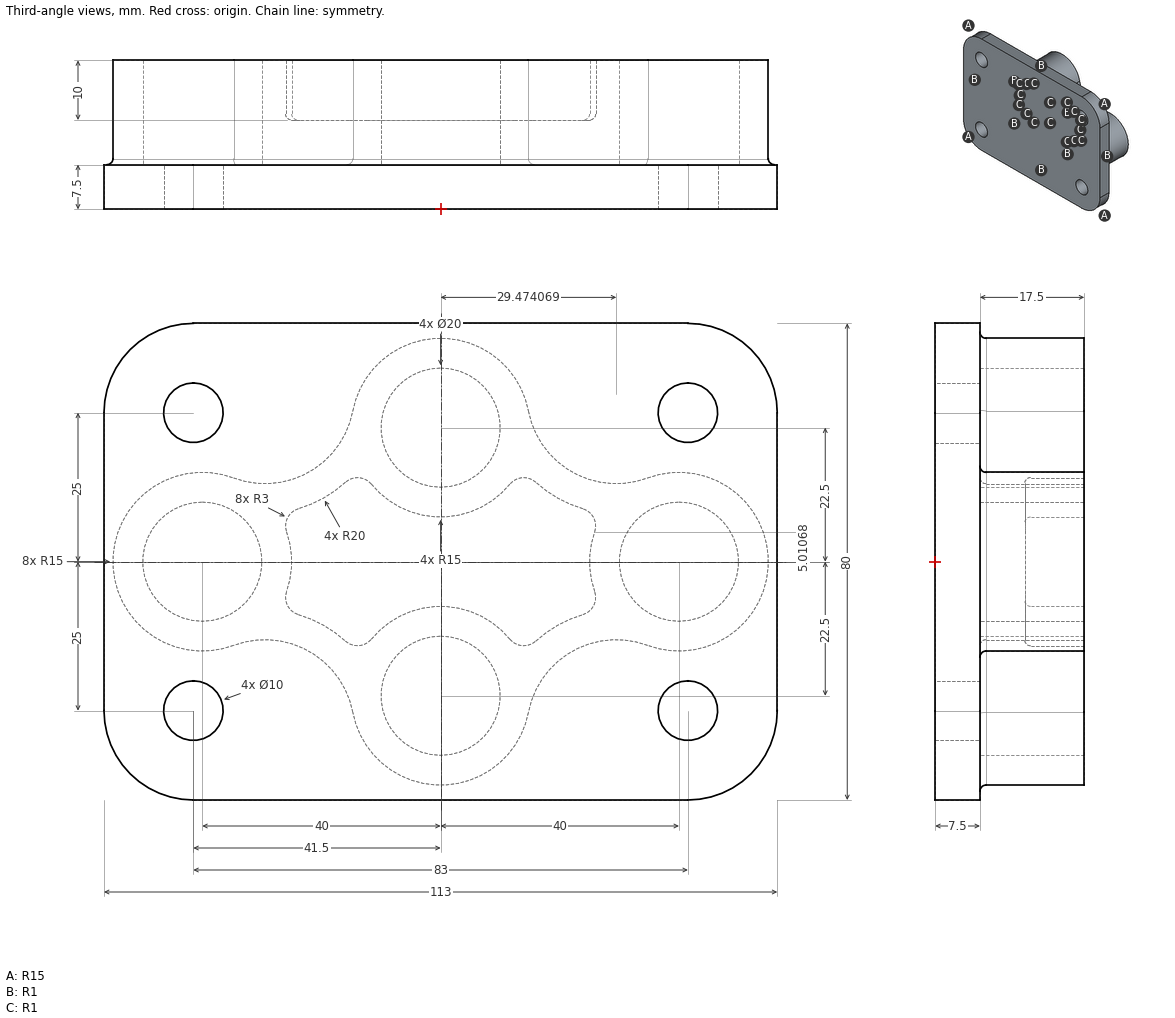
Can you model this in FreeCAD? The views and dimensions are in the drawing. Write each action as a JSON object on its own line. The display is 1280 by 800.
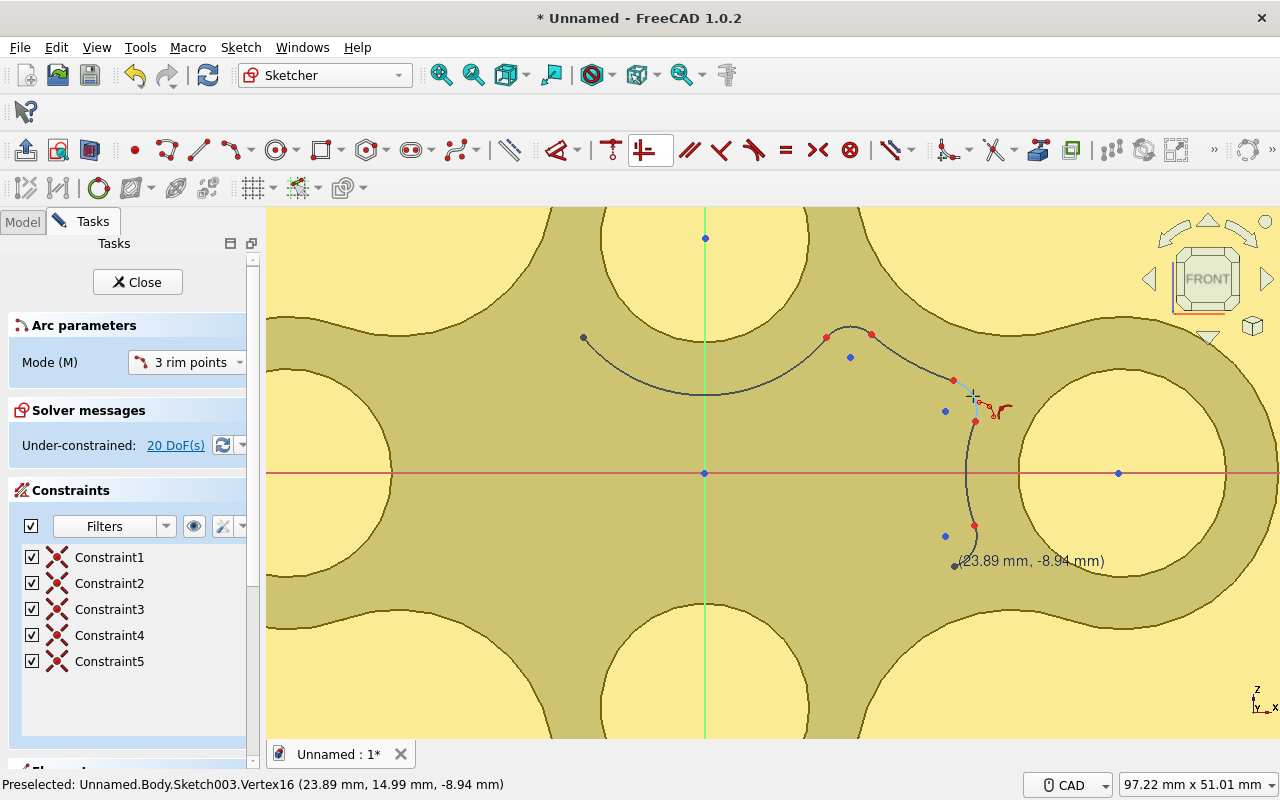
{"action": "left_click", "coordinate": [872, 612]}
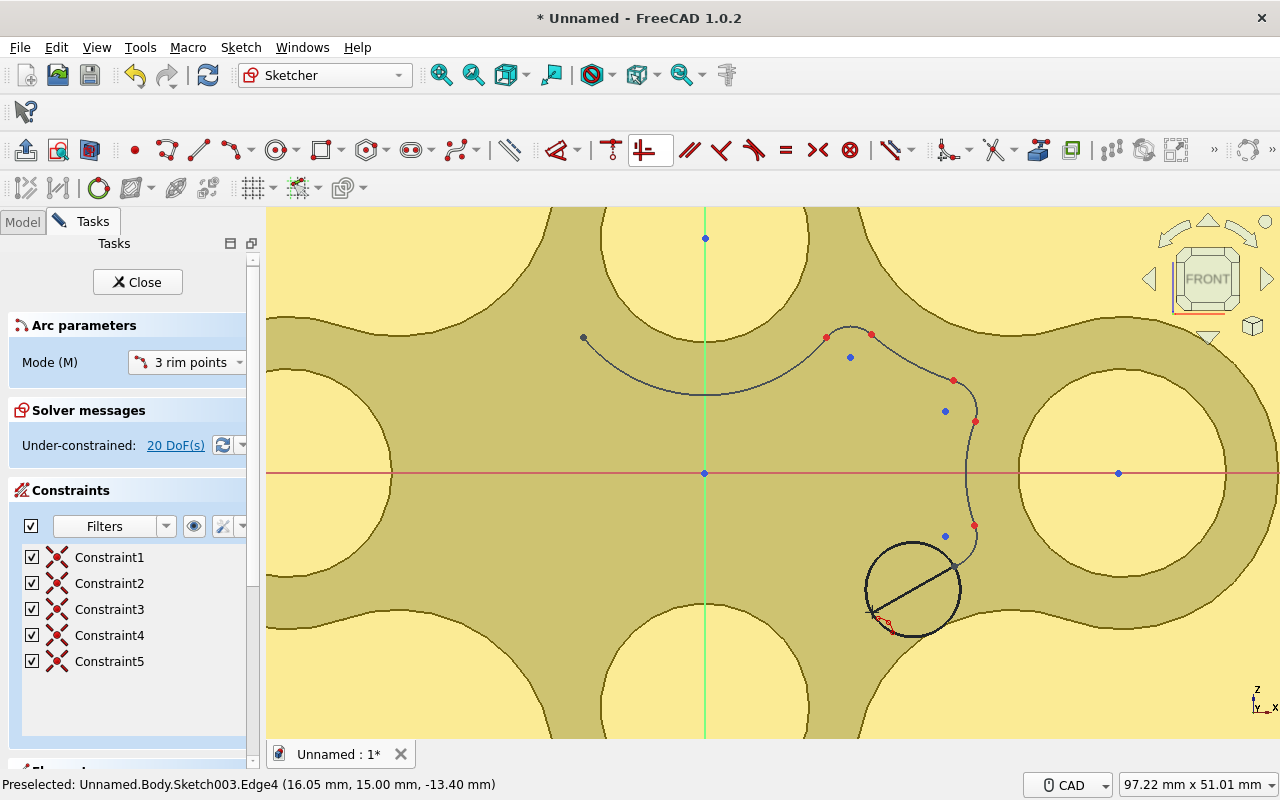
{"action": "scroll", "coordinate": [910, 584], "scroll_direction": "up", "scroll_amount": 6}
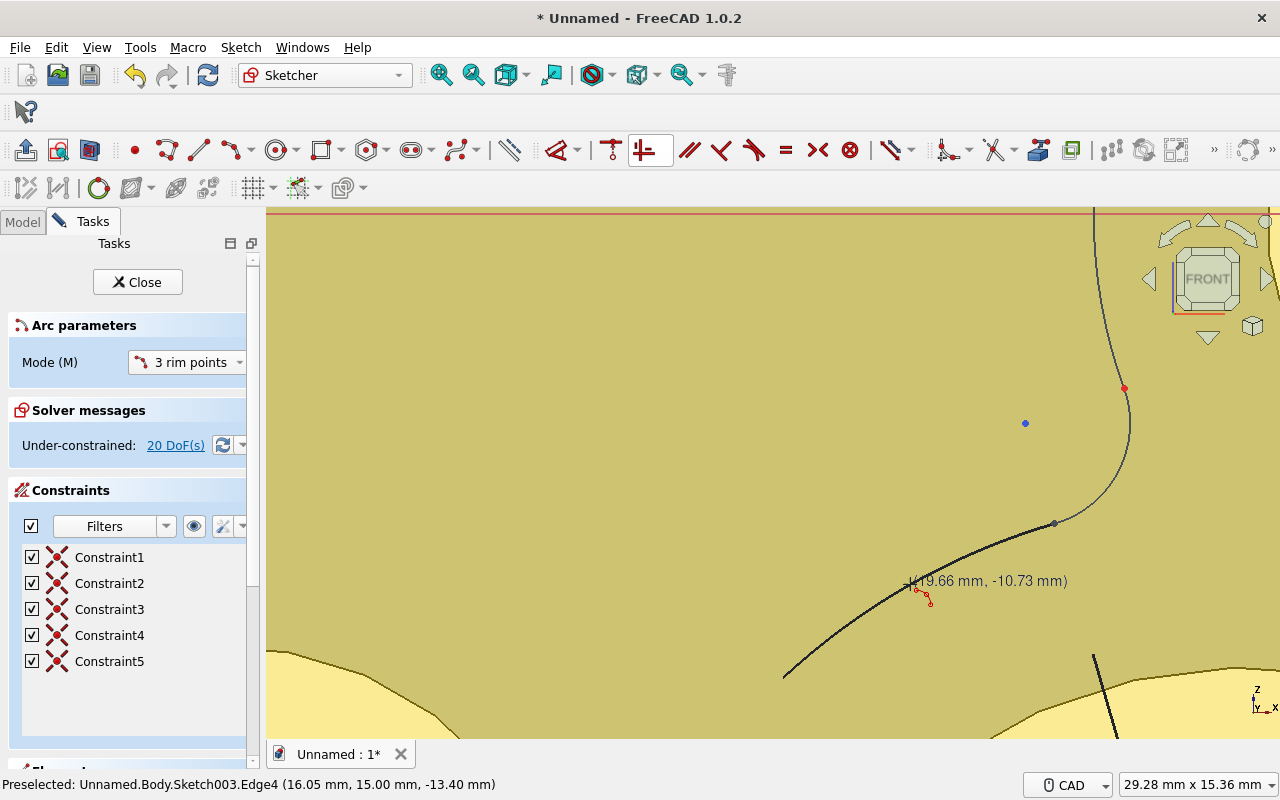
{"action": "left_click", "coordinate": [909, 583]}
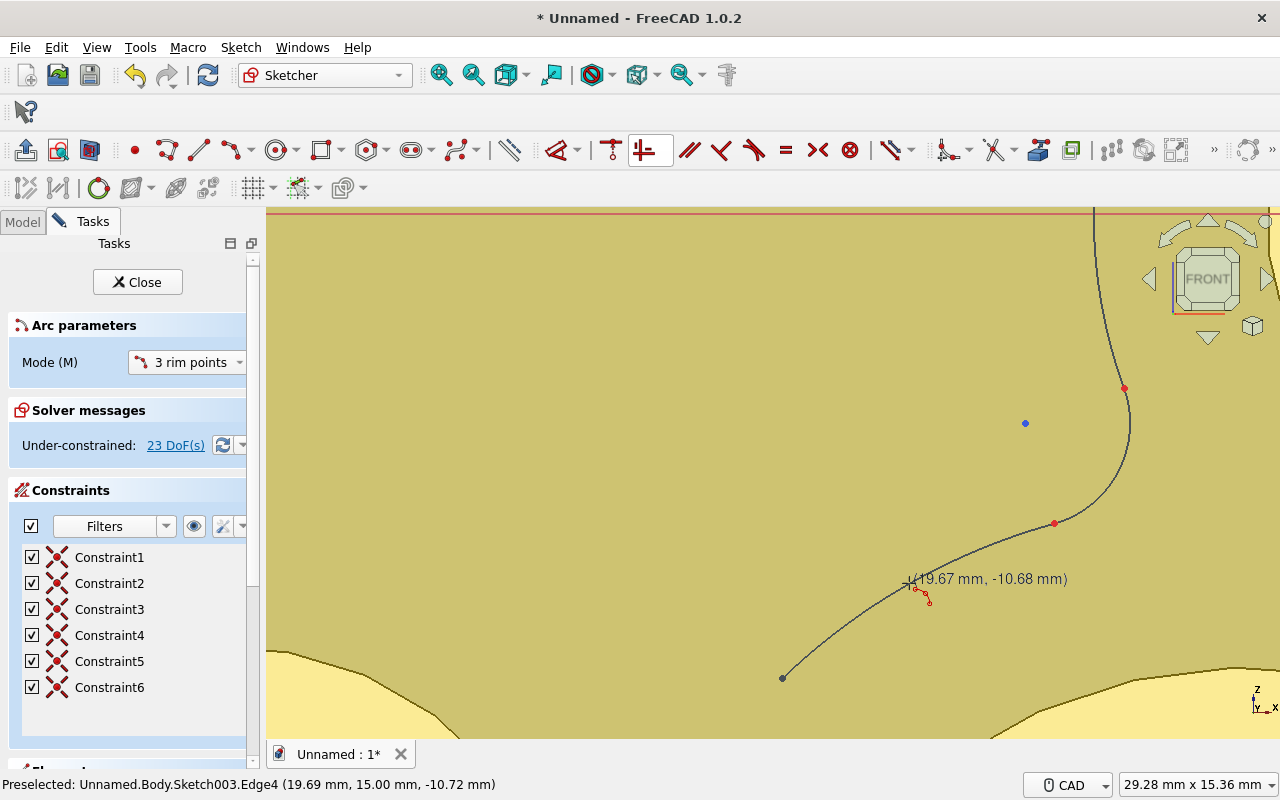
{"action": "left_click", "coordinate": [782, 679]}
{"action": "left_click", "coordinate": [630, 665]}
{"action": "left_click", "coordinate": [703, 703]}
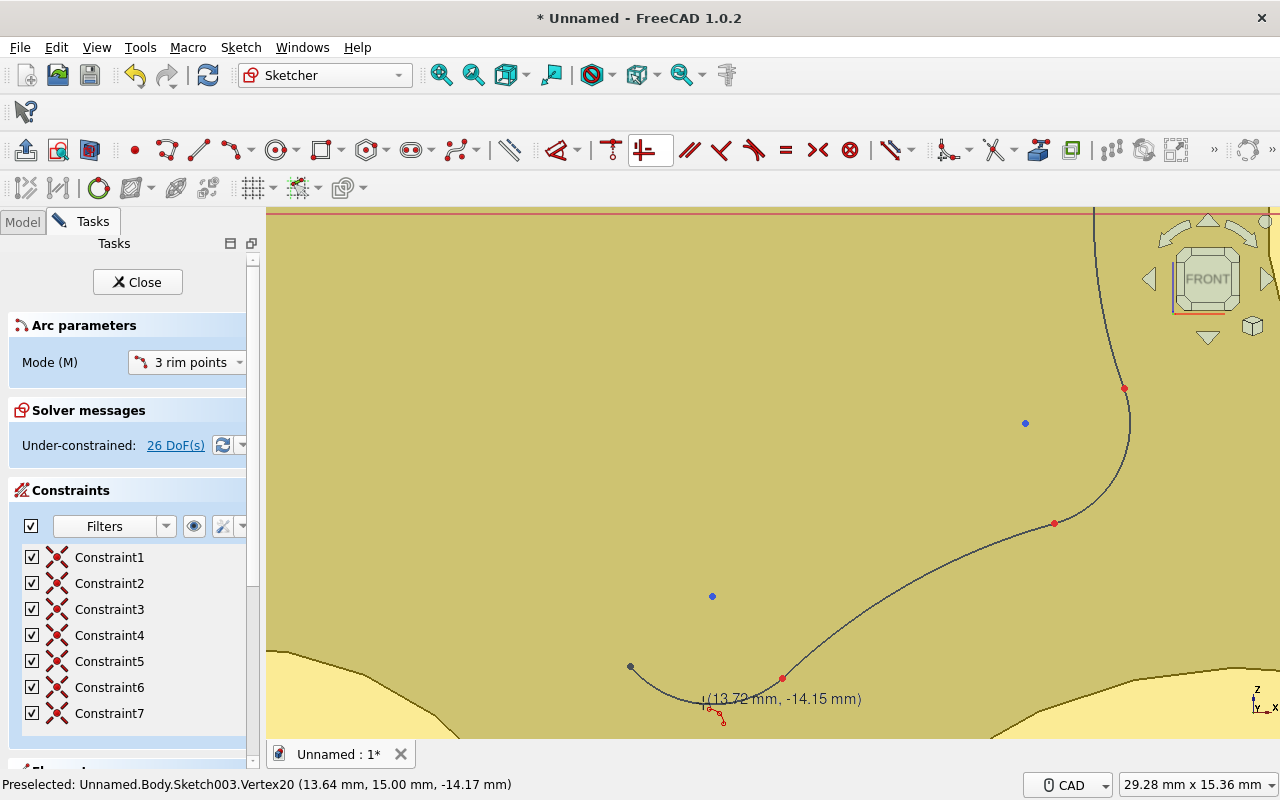
{"action": "left_click", "coordinate": [630, 666]}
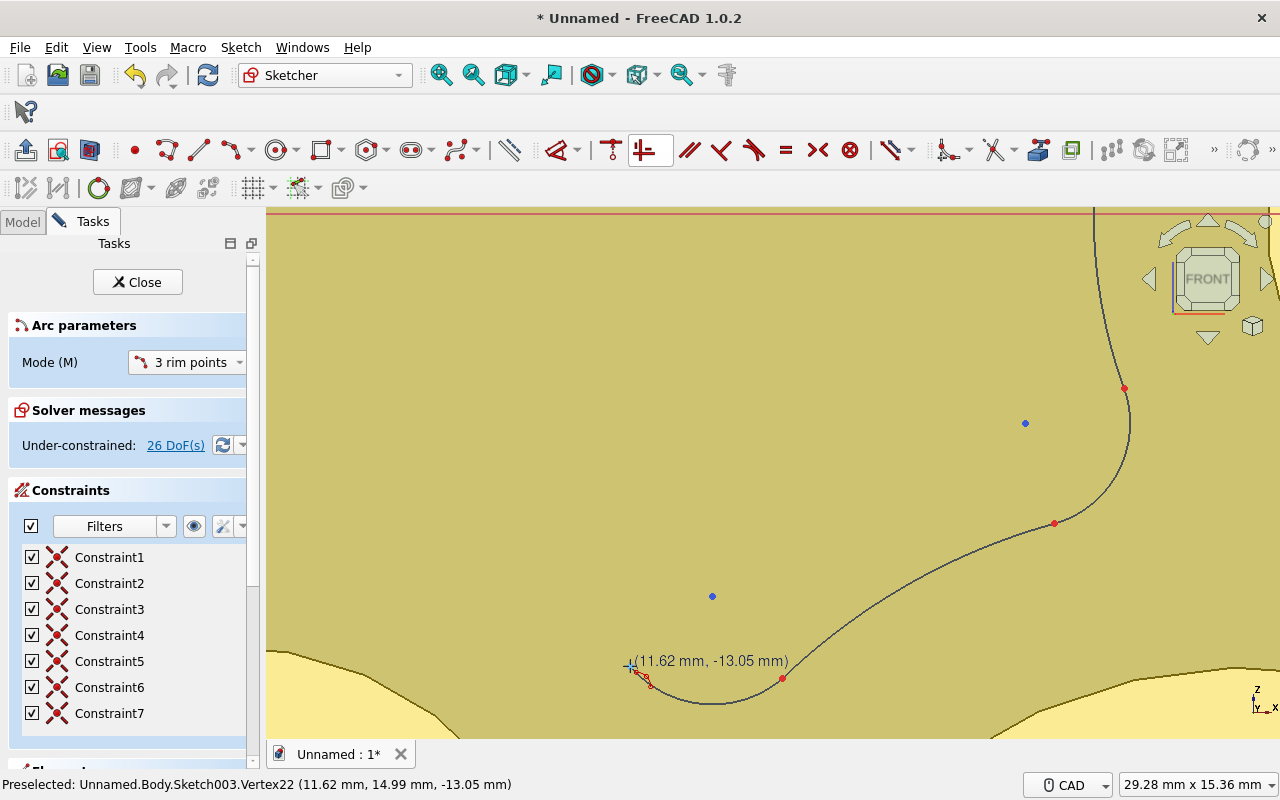
{"action": "scroll", "coordinate": [910, 585], "scroll_direction": "down", "scroll_amount": 6}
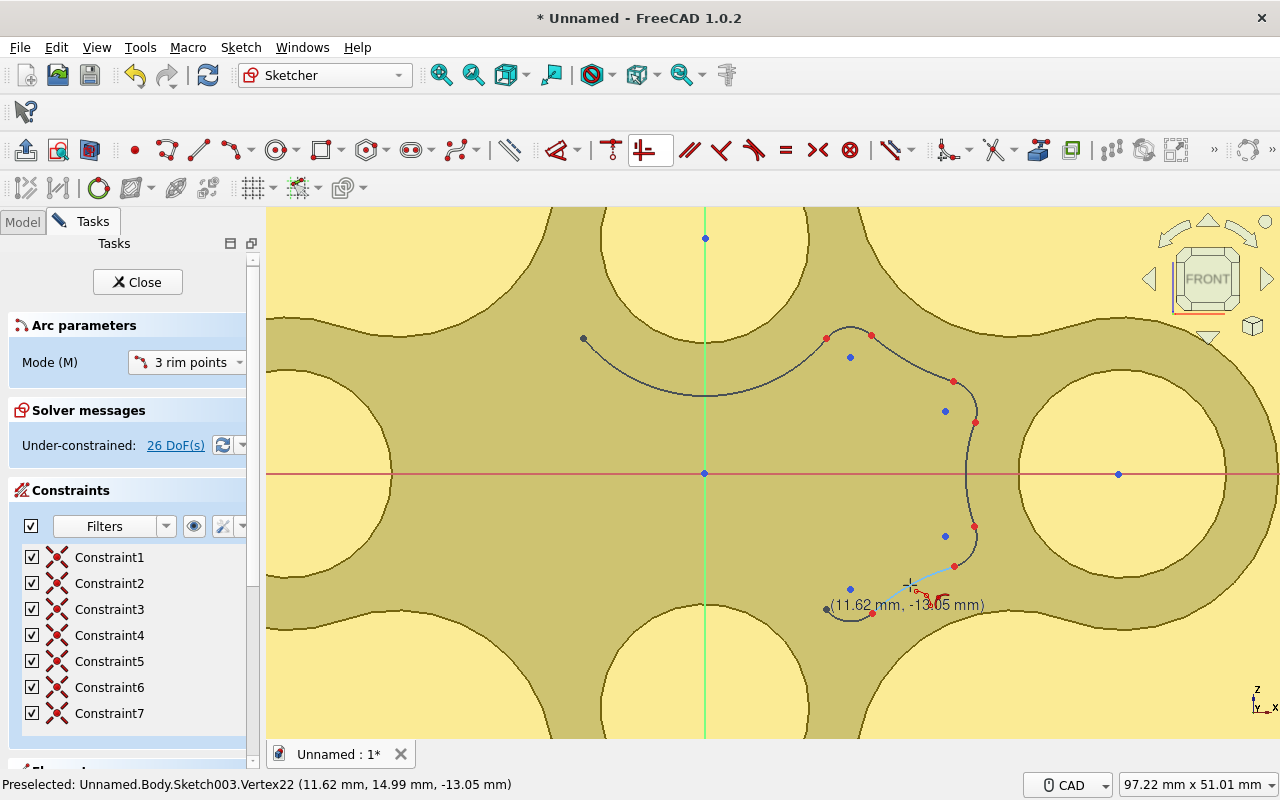
{"action": "left_click", "coordinate": [584, 610]}
{"action": "left_click", "coordinate": [733, 554]}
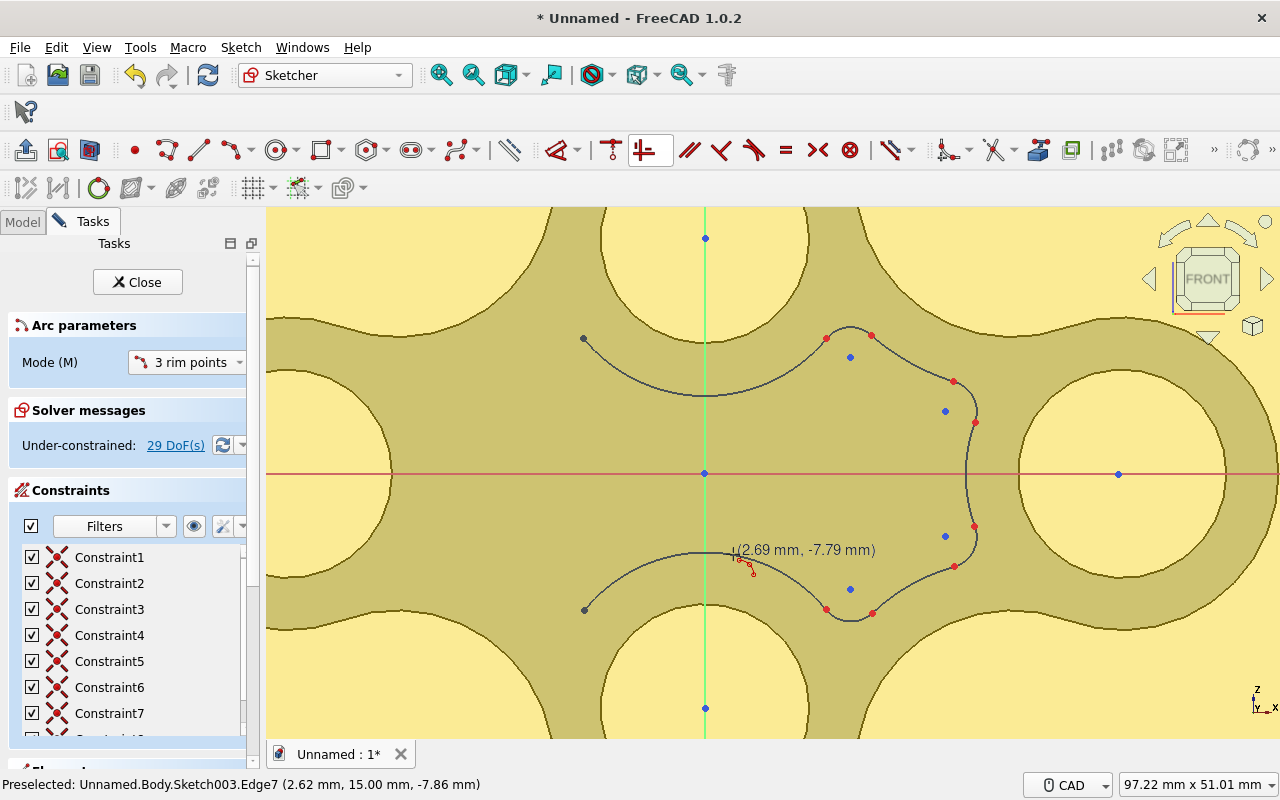
{"action": "left_click", "coordinate": [584, 611]}
{"action": "left_click", "coordinate": [538, 613]}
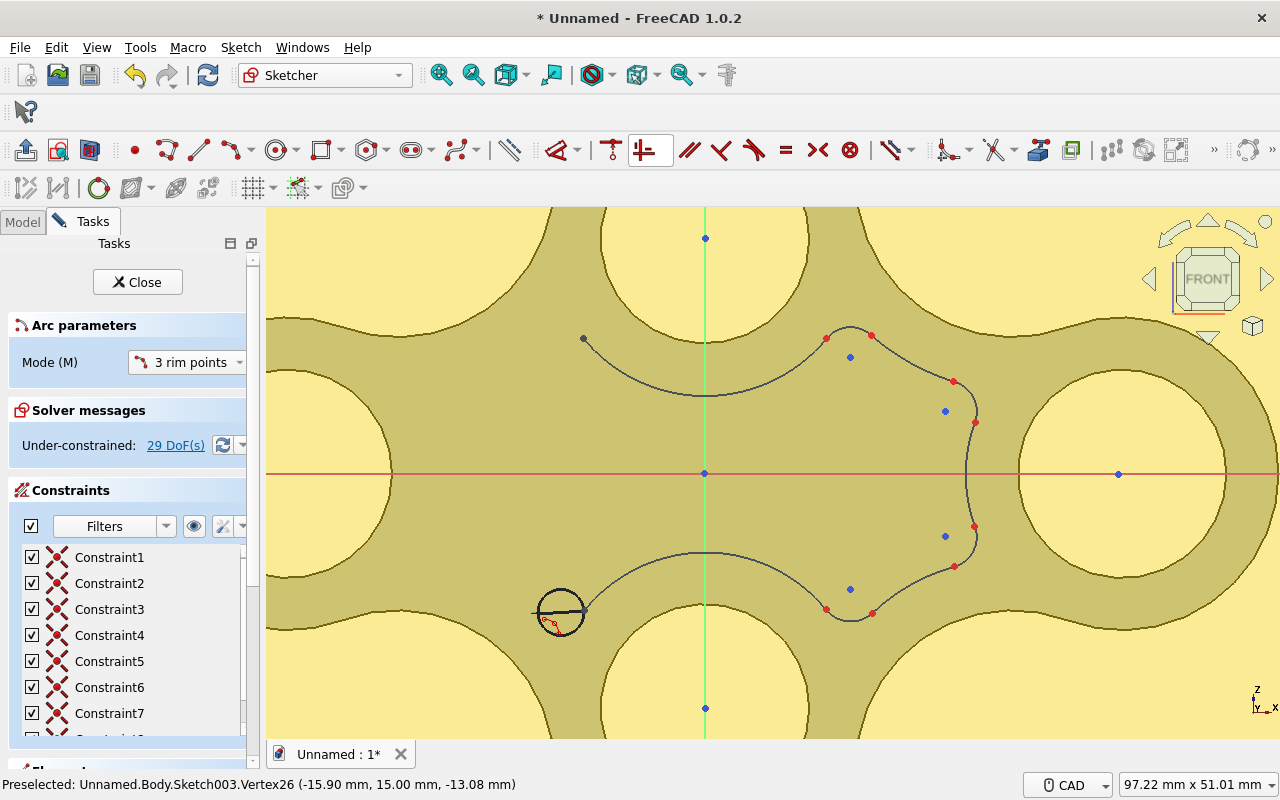
{"action": "scroll", "coordinate": [562, 621], "scroll_direction": "up", "scroll_amount": 3}